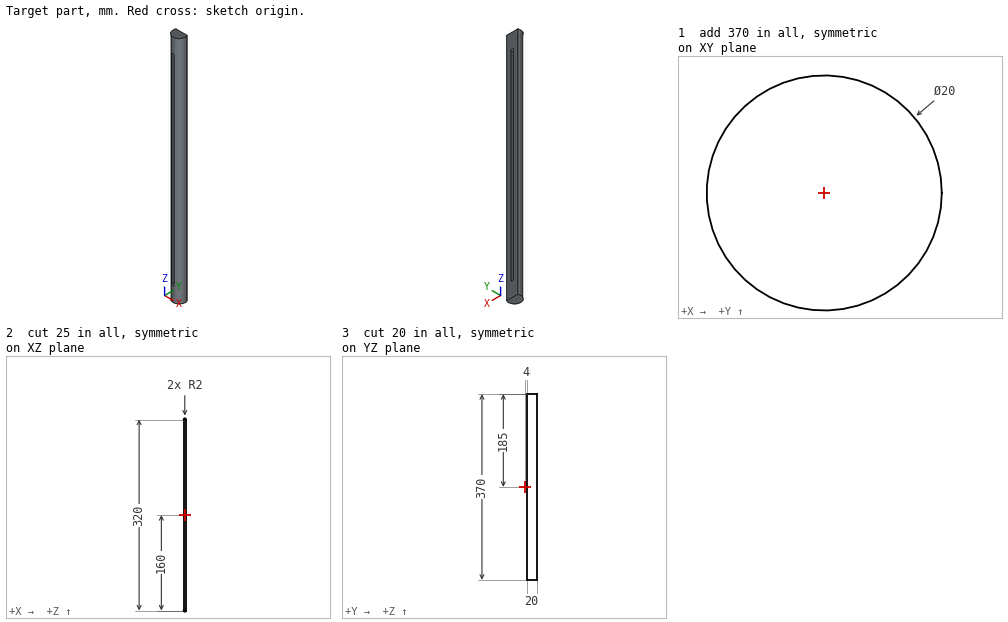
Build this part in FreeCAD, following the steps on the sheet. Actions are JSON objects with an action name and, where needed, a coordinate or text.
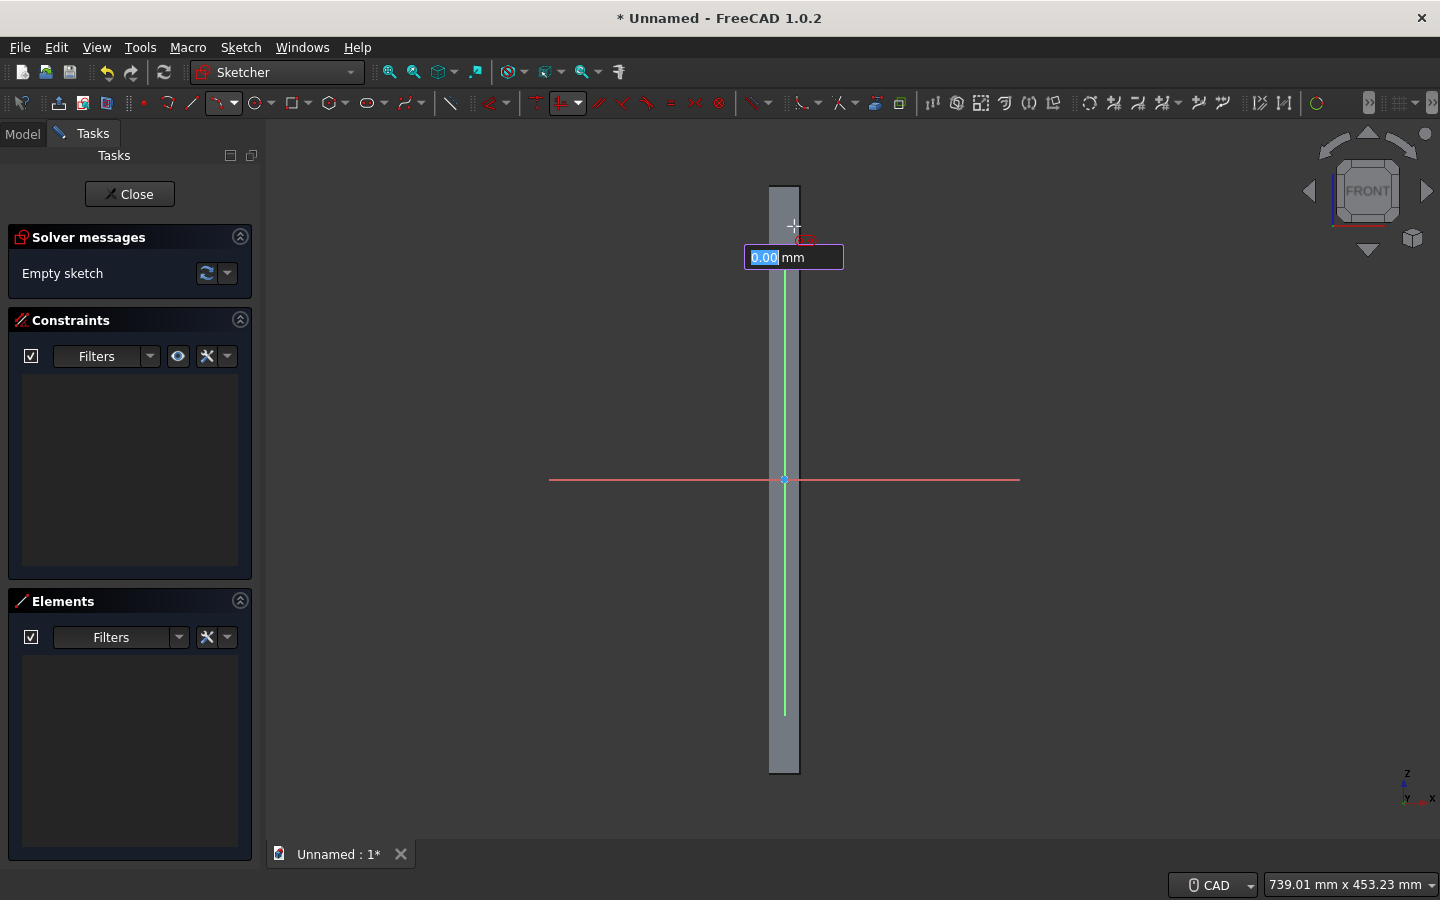
{"action": "scroll", "coordinate": [781, 556], "scroll_direction": "up", "scroll_amount": 9}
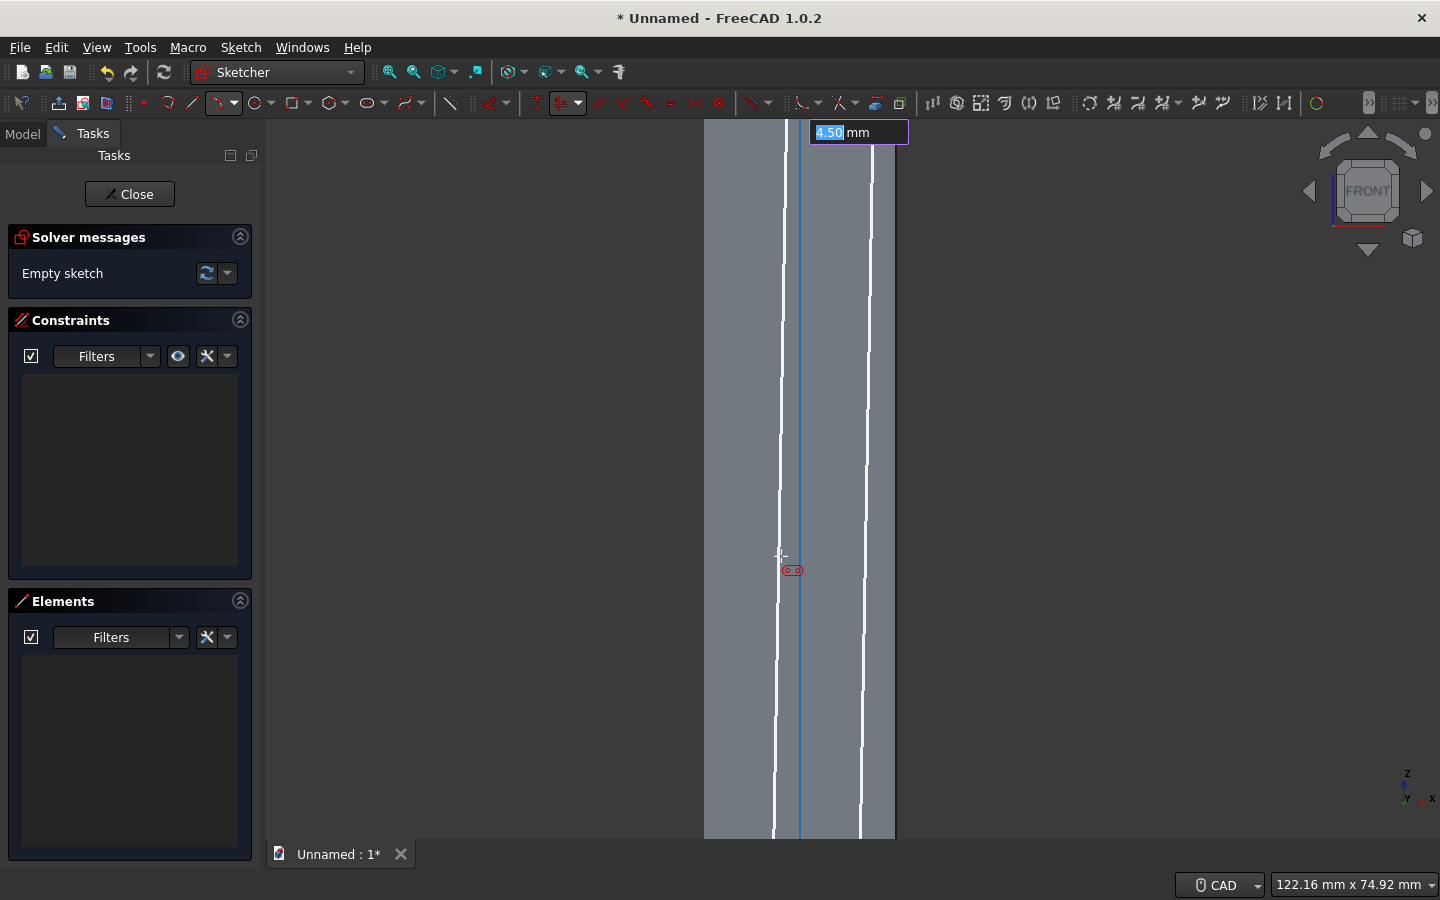
{"action": "left_click", "coordinate": [781, 554]}
{"action": "key", "text": "Escape"}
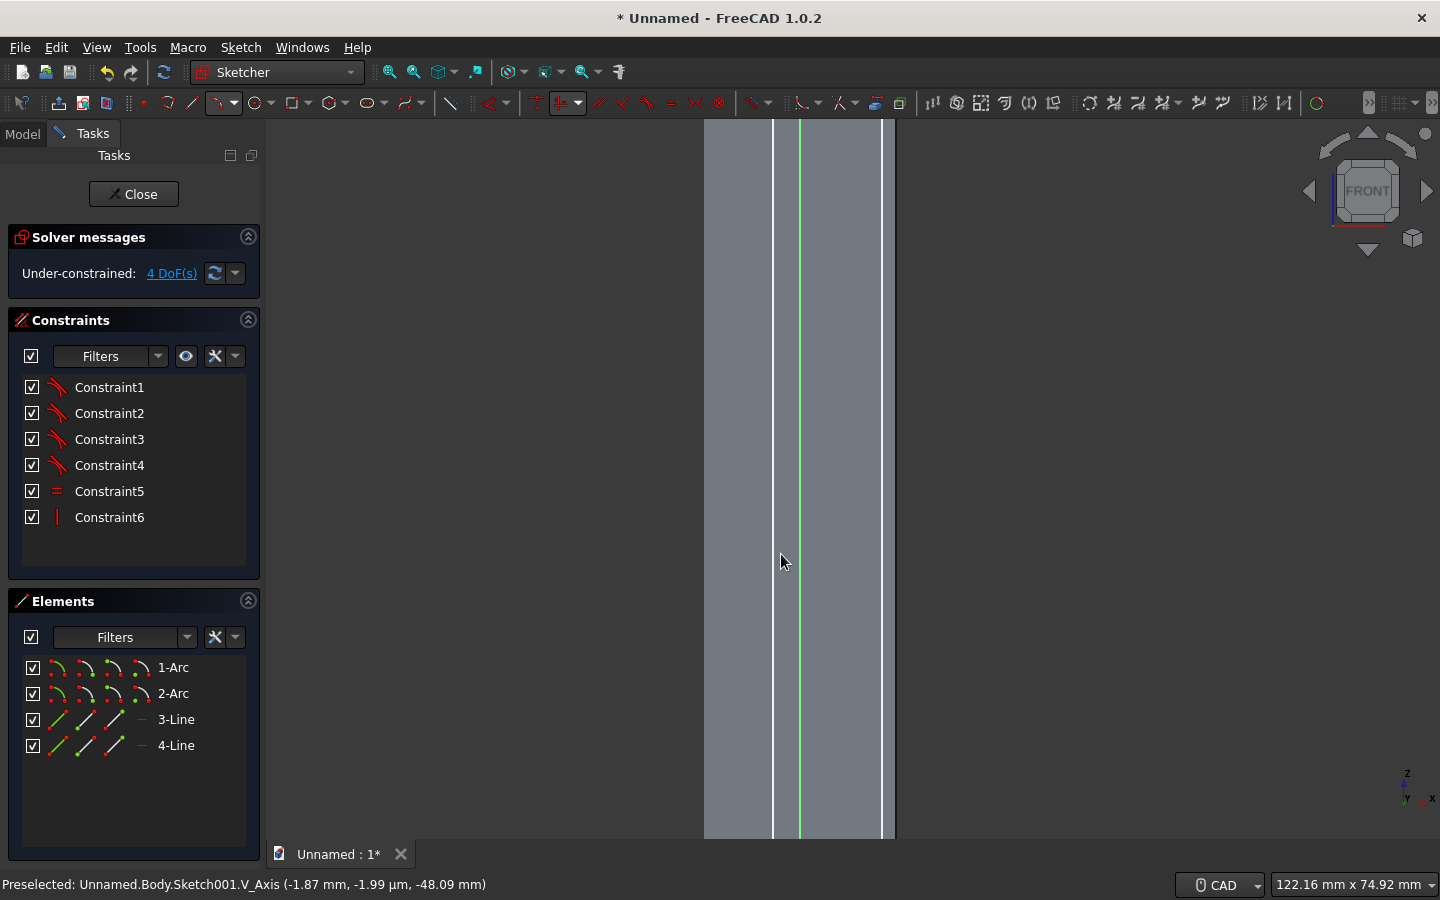
{"action": "scroll", "coordinate": [781, 555], "scroll_direction": "down", "scroll_amount": 9}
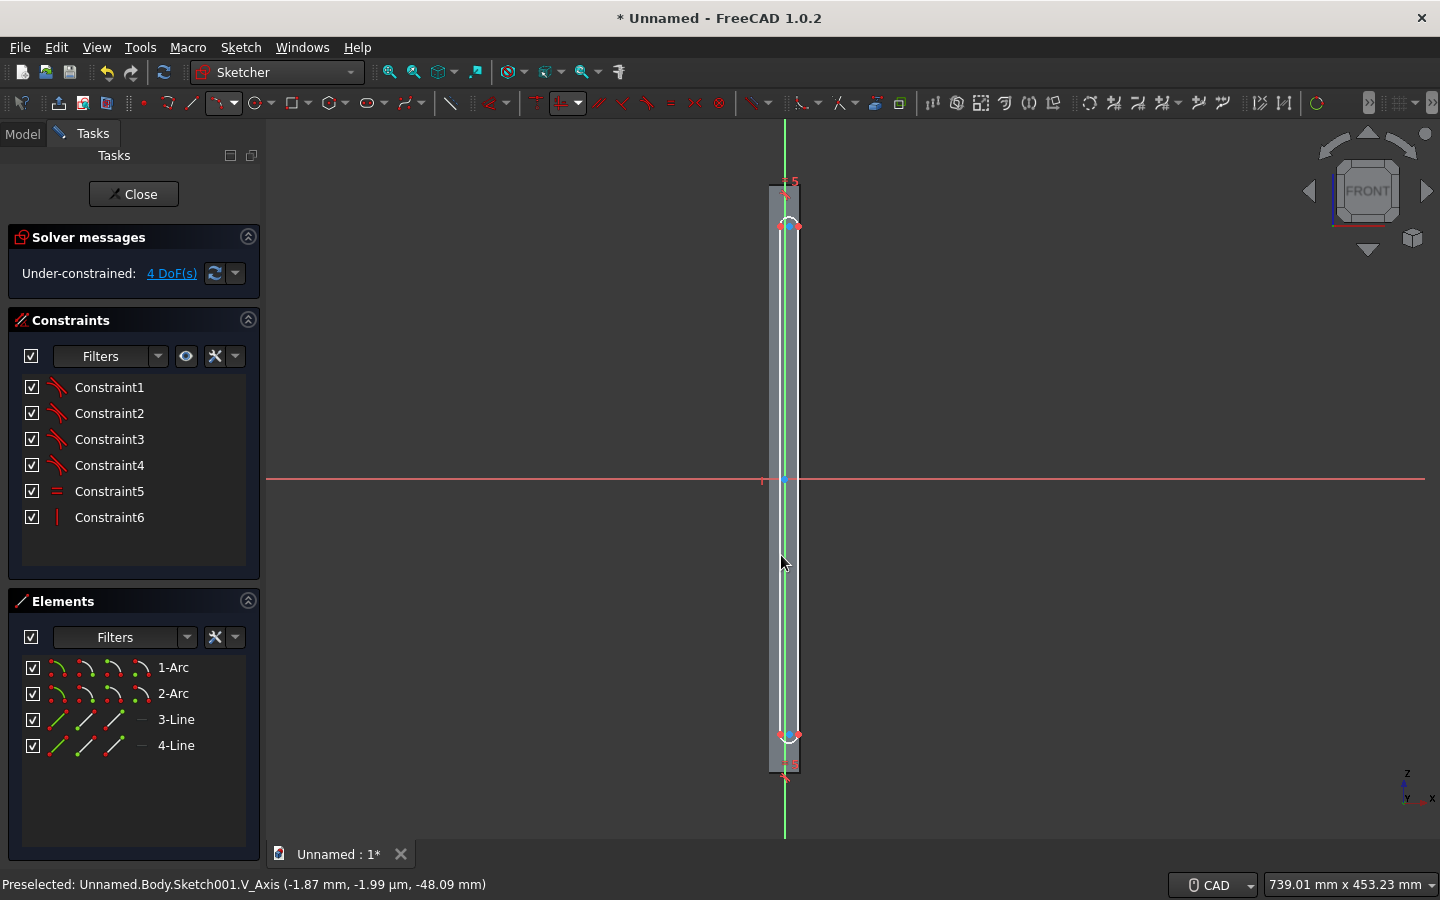
{"action": "scroll", "coordinate": [789, 734], "scroll_direction": "up", "scroll_amount": 2}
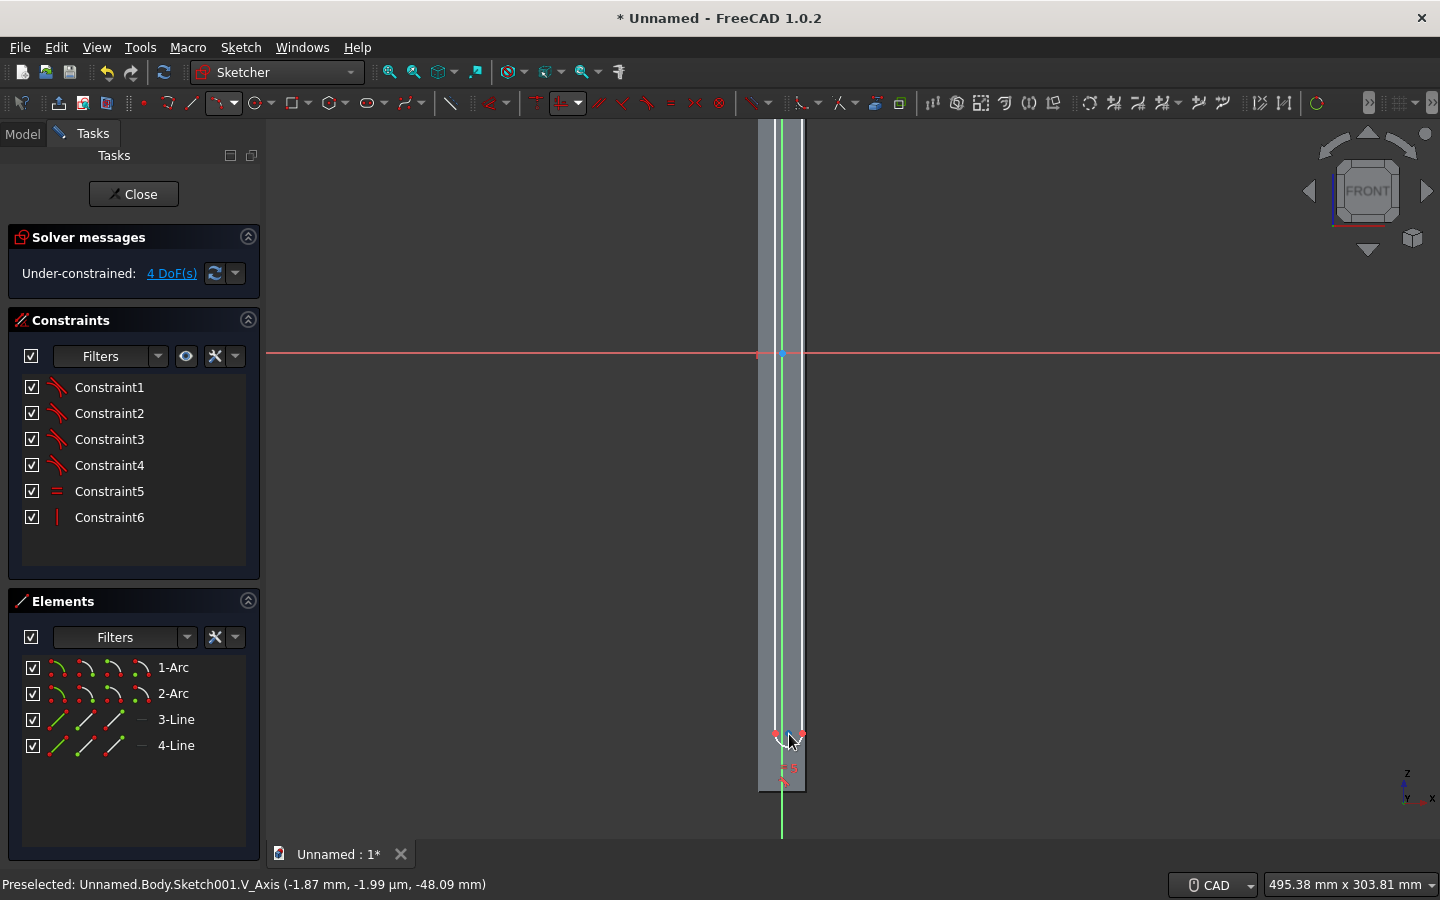
{"action": "left_click", "coordinate": [789, 734]}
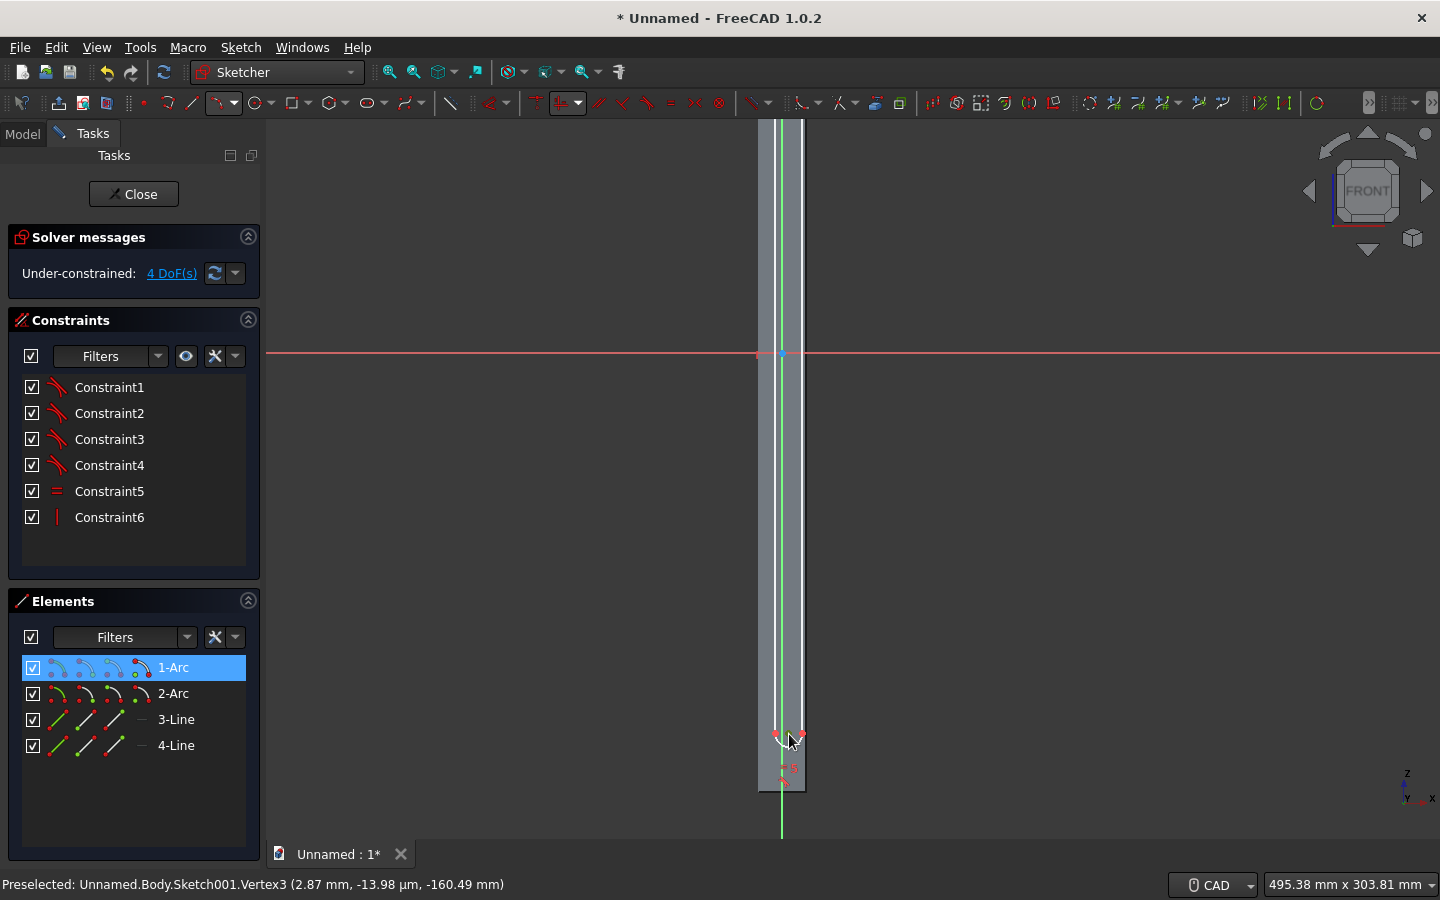
{"action": "left_click", "coordinate": [782, 716]}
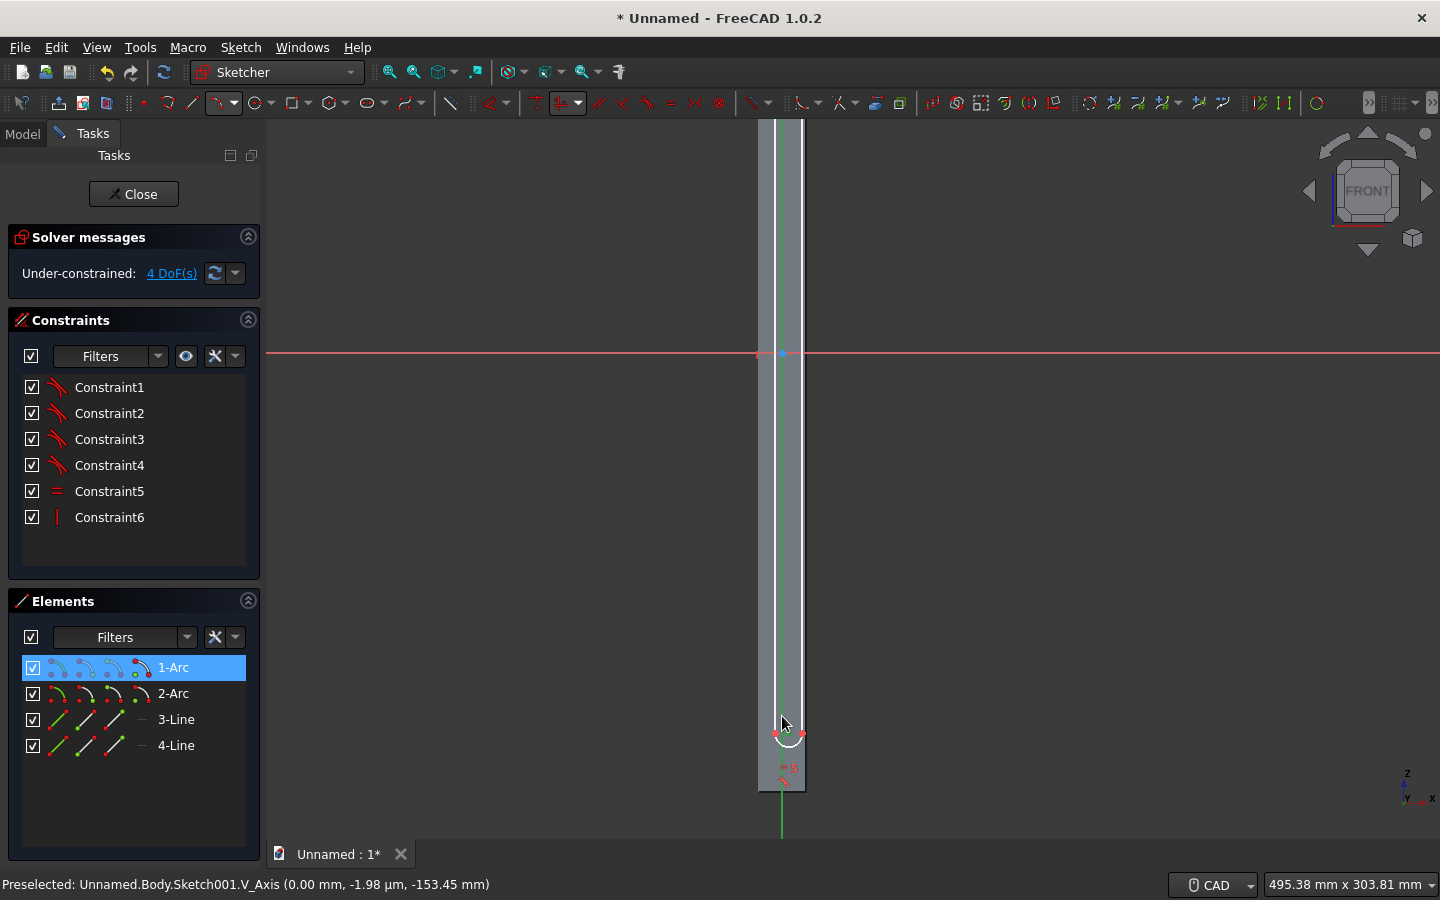
{"action": "left_click", "coordinate": [536, 104]}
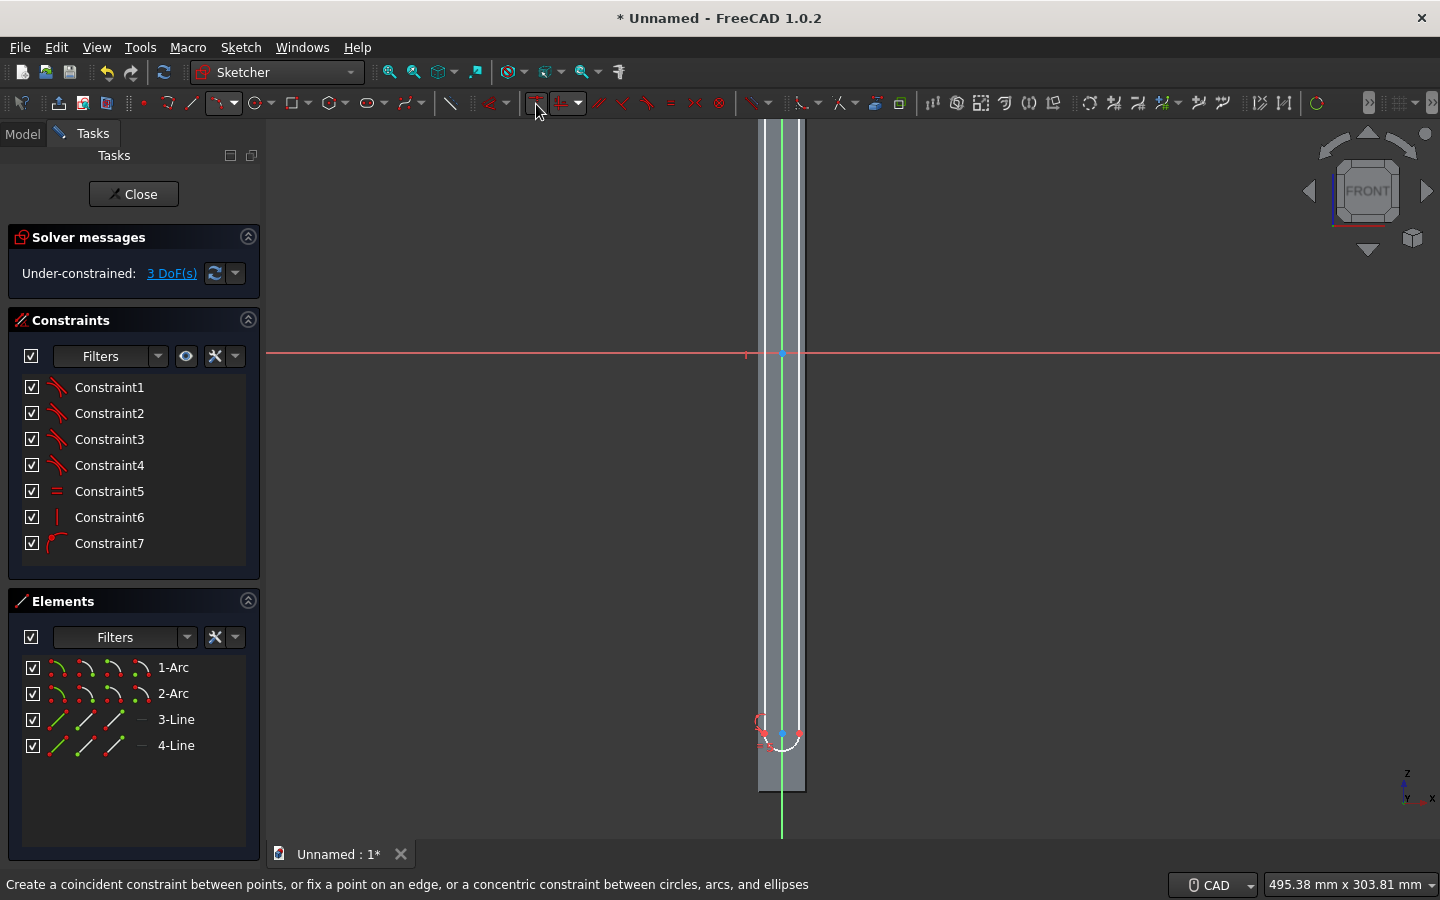
{"action": "left_click", "coordinate": [490, 104]}